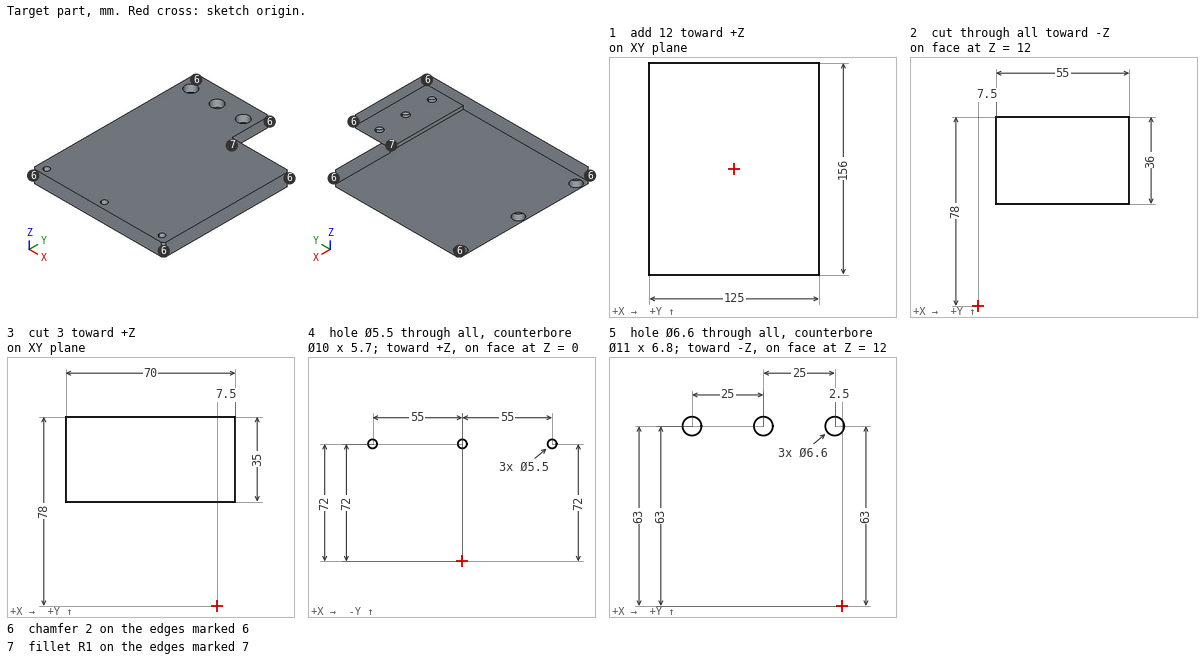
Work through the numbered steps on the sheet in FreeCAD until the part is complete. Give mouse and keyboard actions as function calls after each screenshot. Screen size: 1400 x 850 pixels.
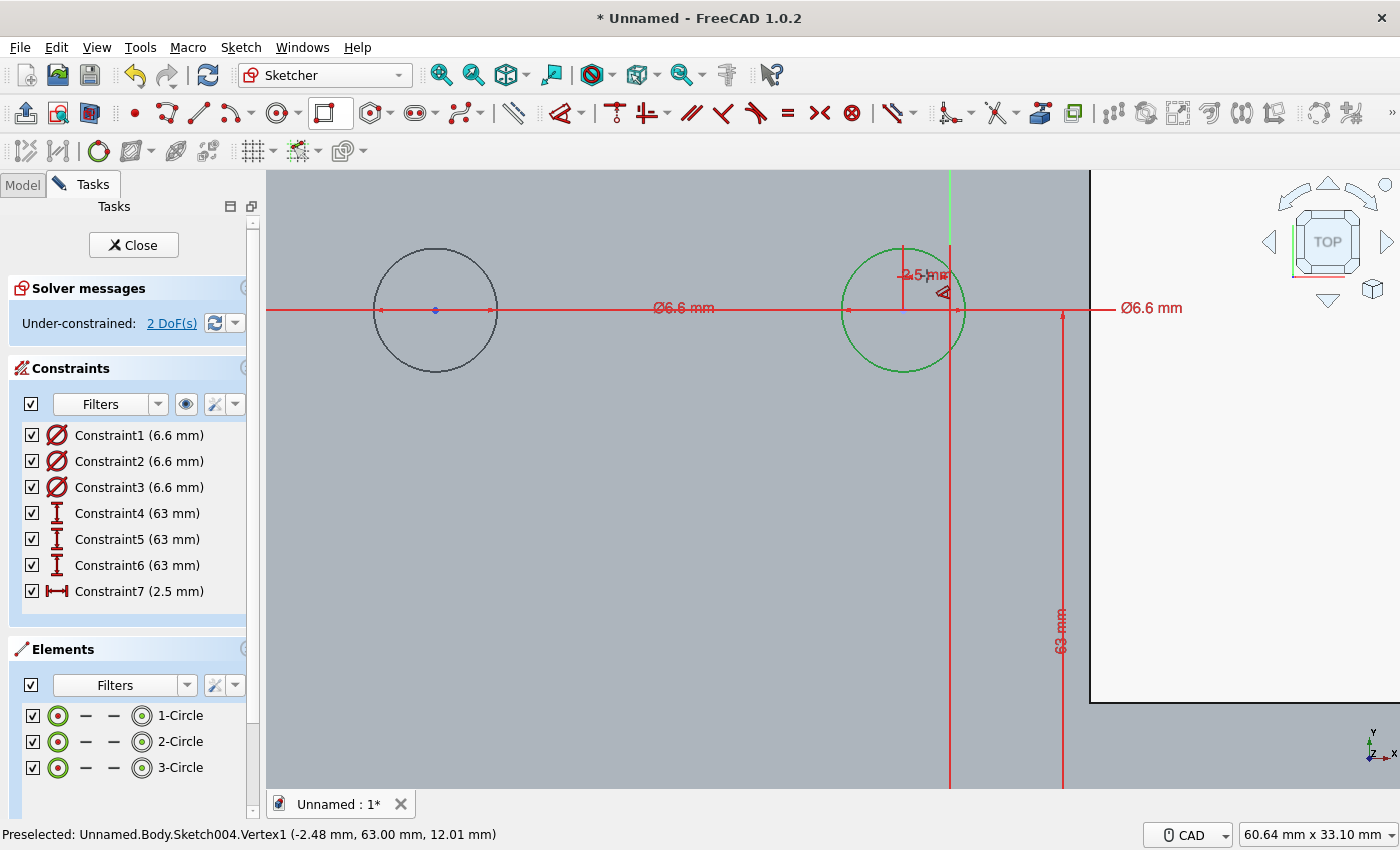
click(903, 310)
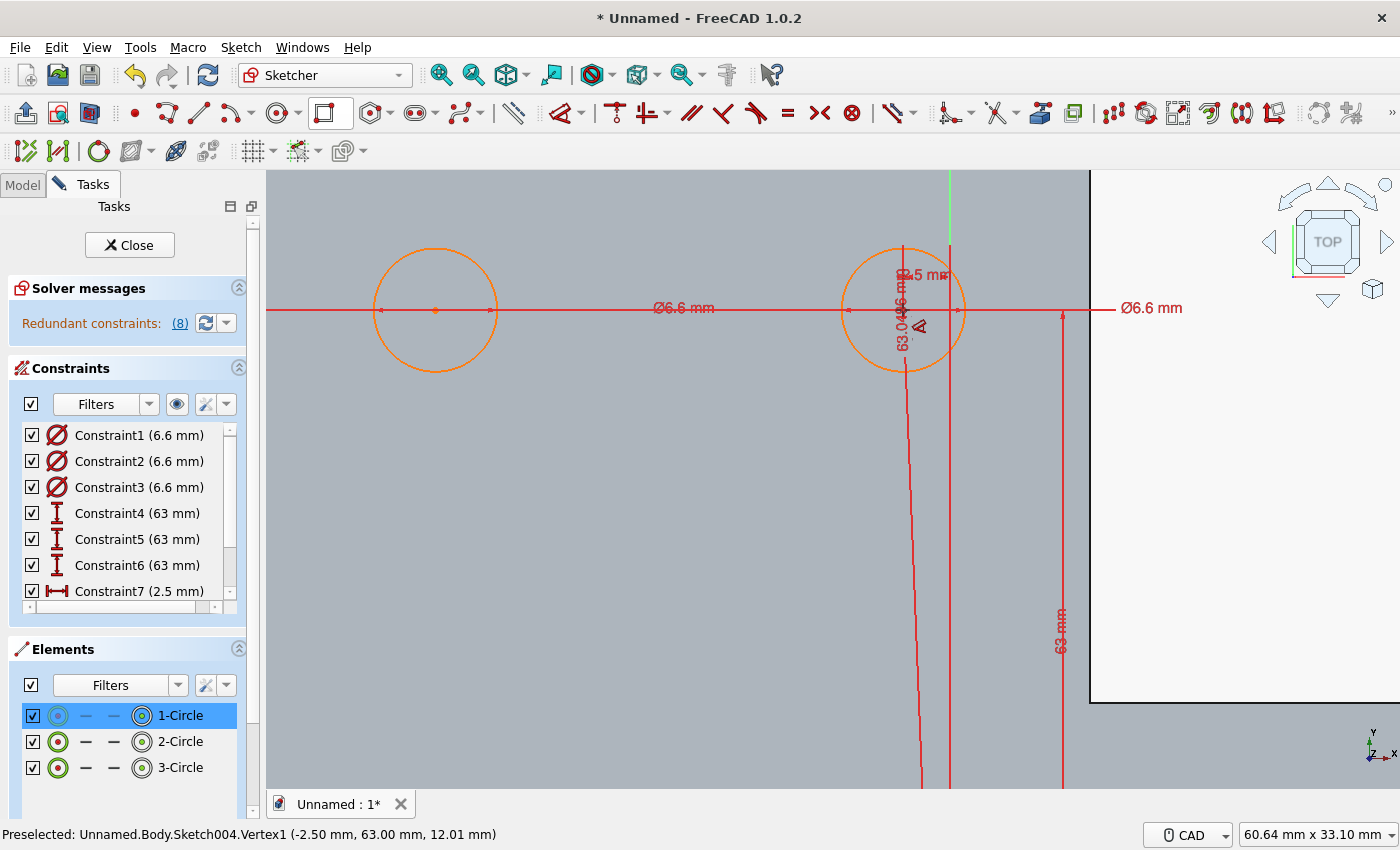
click(436, 310)
click(669, 276)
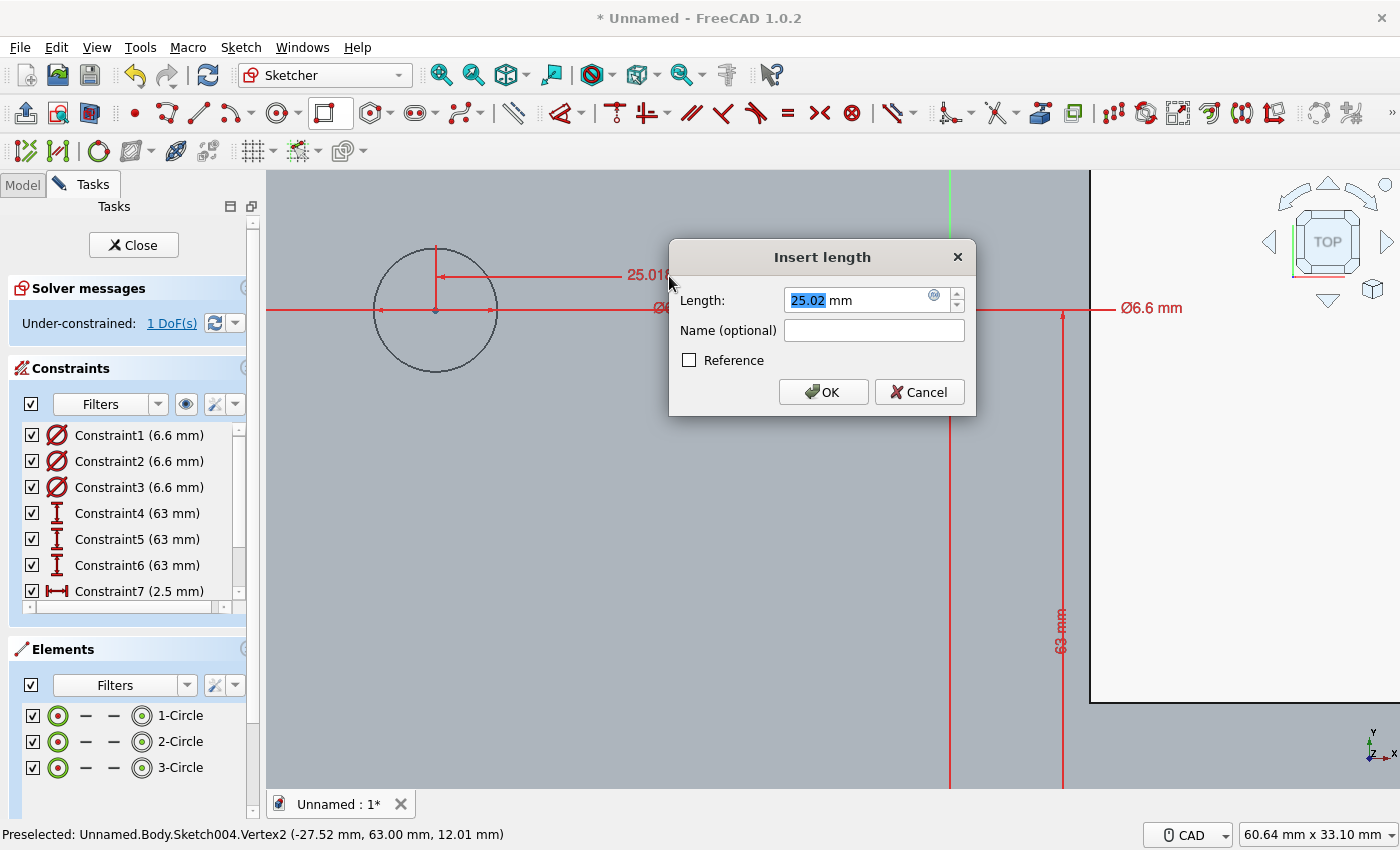
text(25)
key(Return)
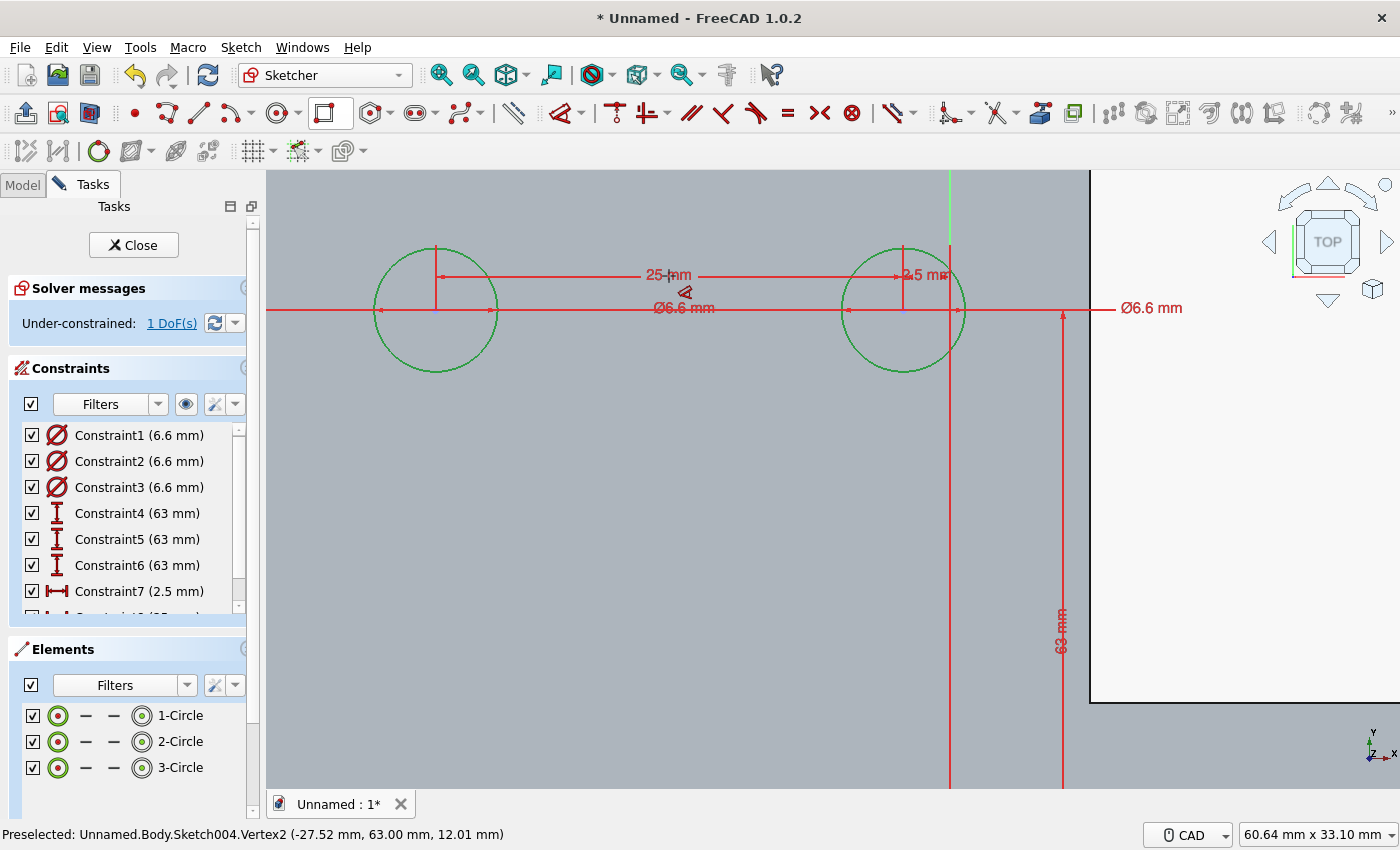
click(436, 310)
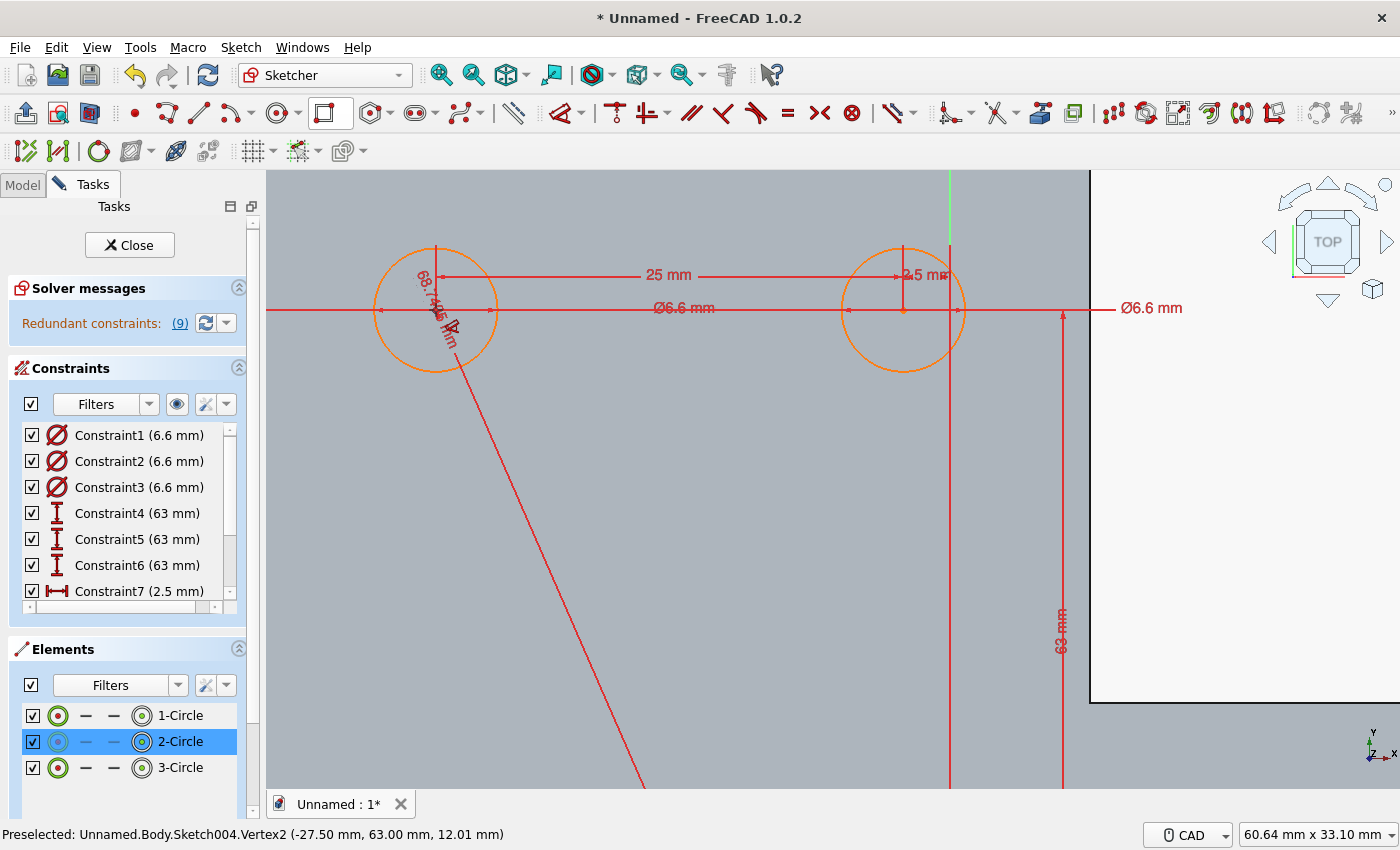
scroll(906, 312, down, 6)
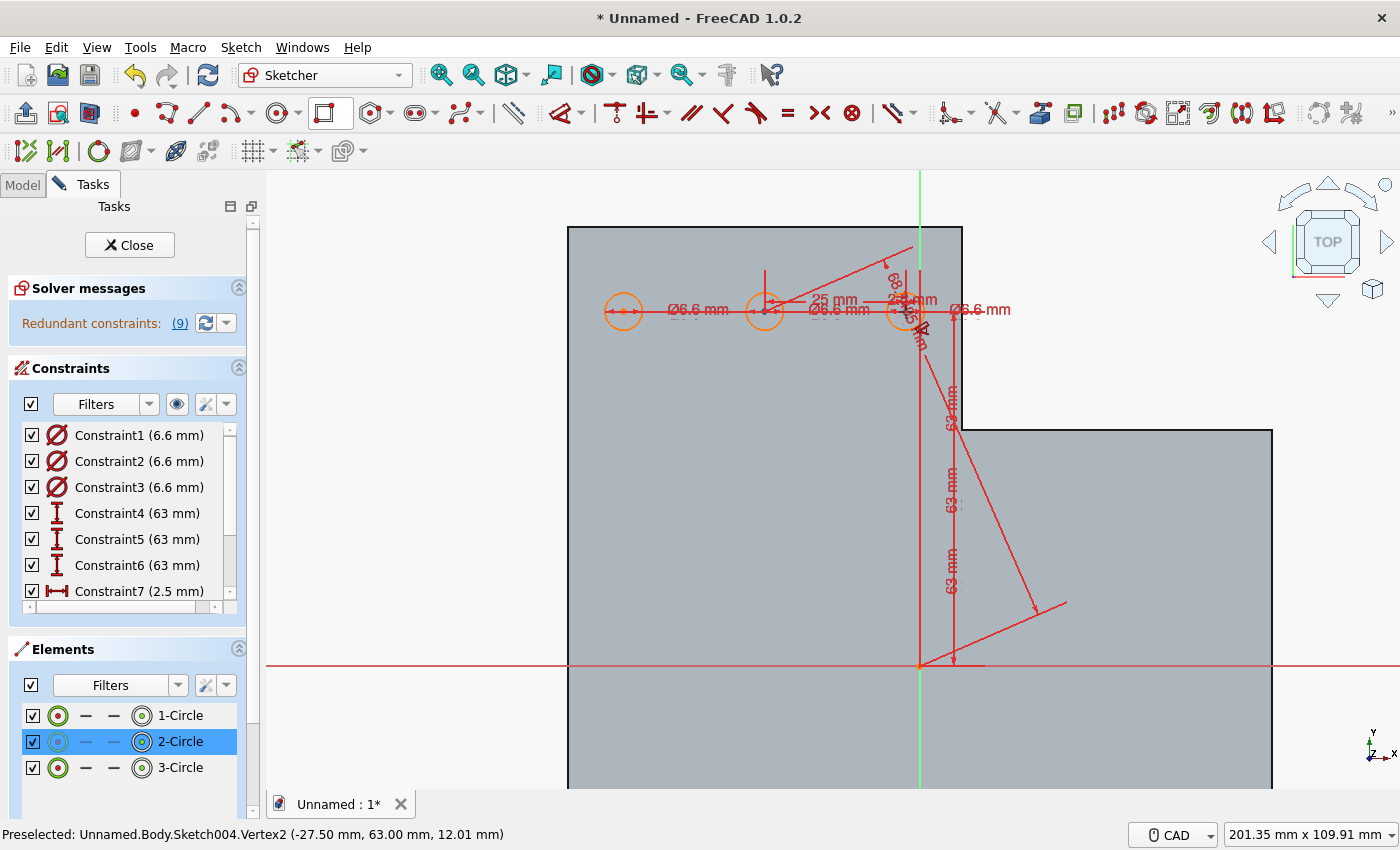
click(624, 312)
click(694, 278)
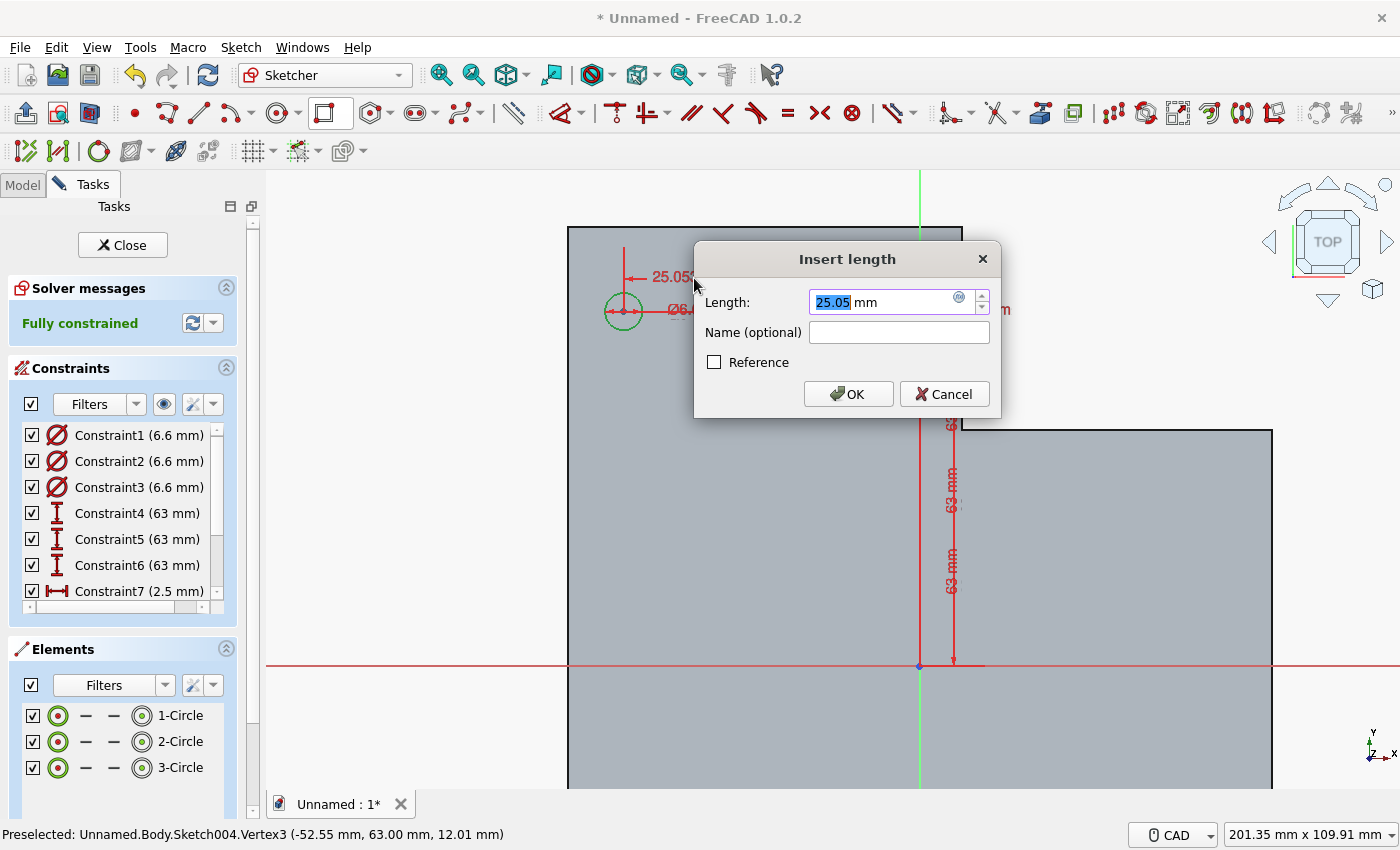
text(25)
key(Return)
key(Escape)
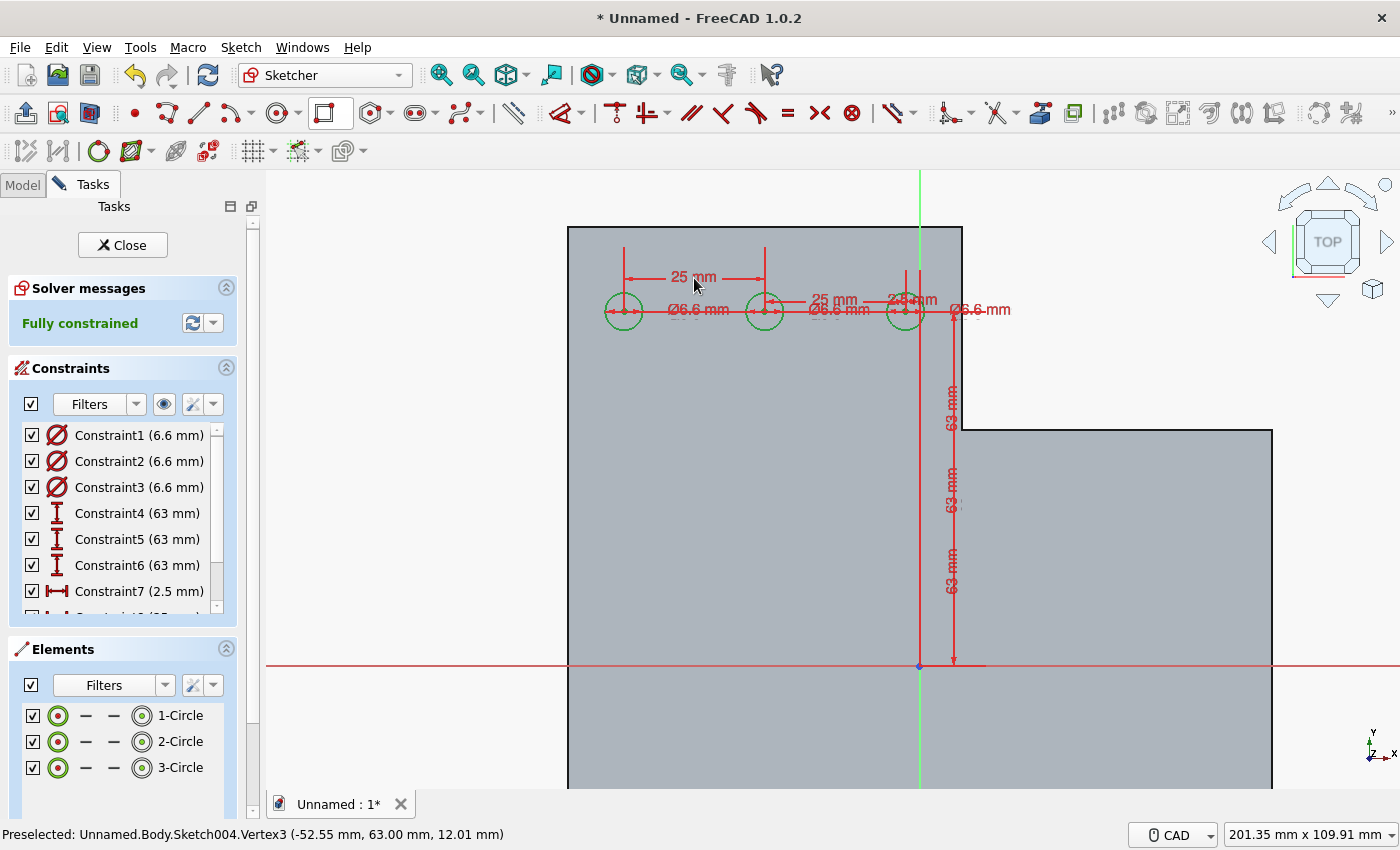
click(123, 245)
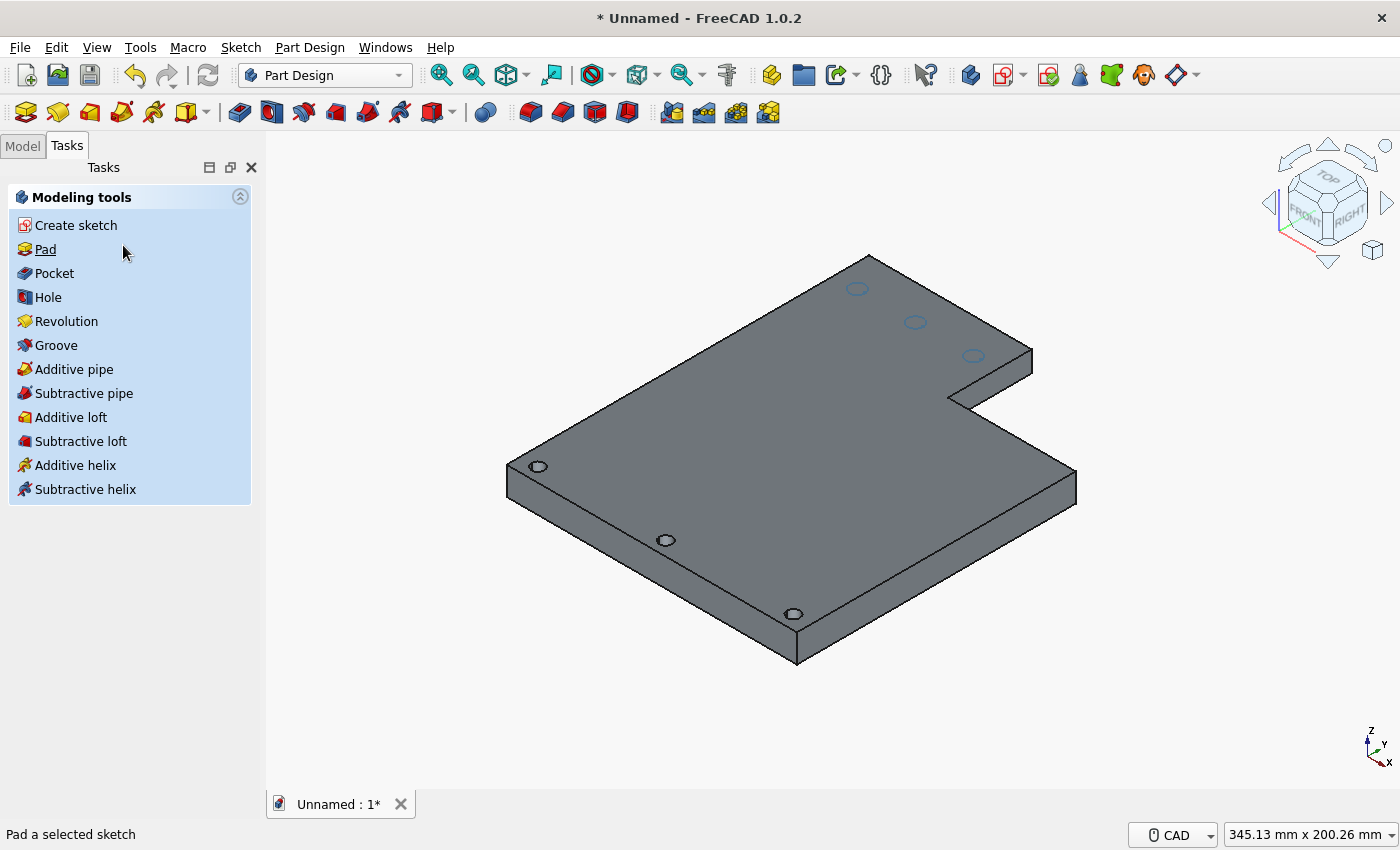
click(272, 112)